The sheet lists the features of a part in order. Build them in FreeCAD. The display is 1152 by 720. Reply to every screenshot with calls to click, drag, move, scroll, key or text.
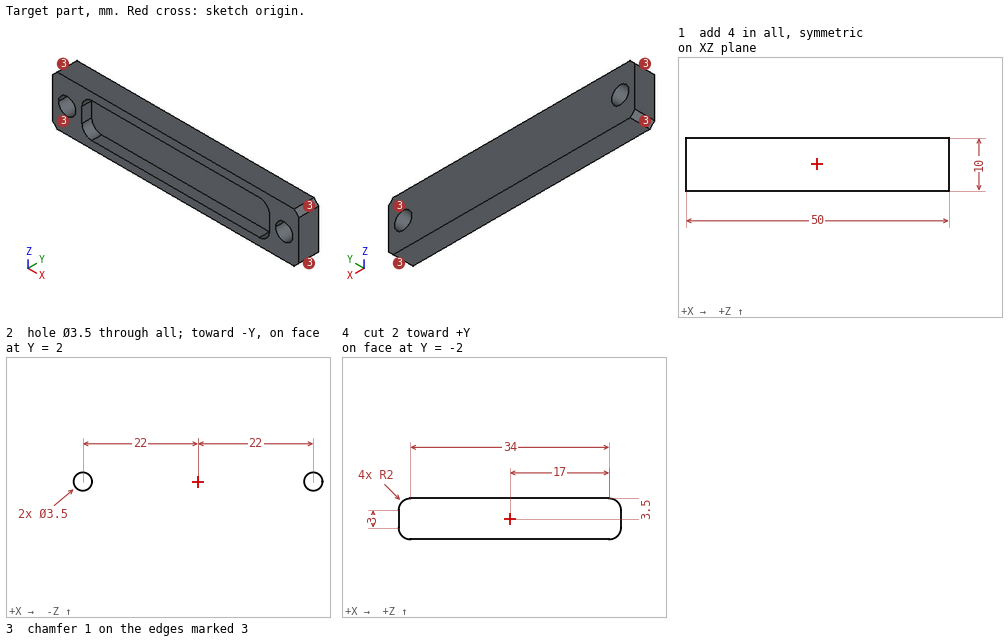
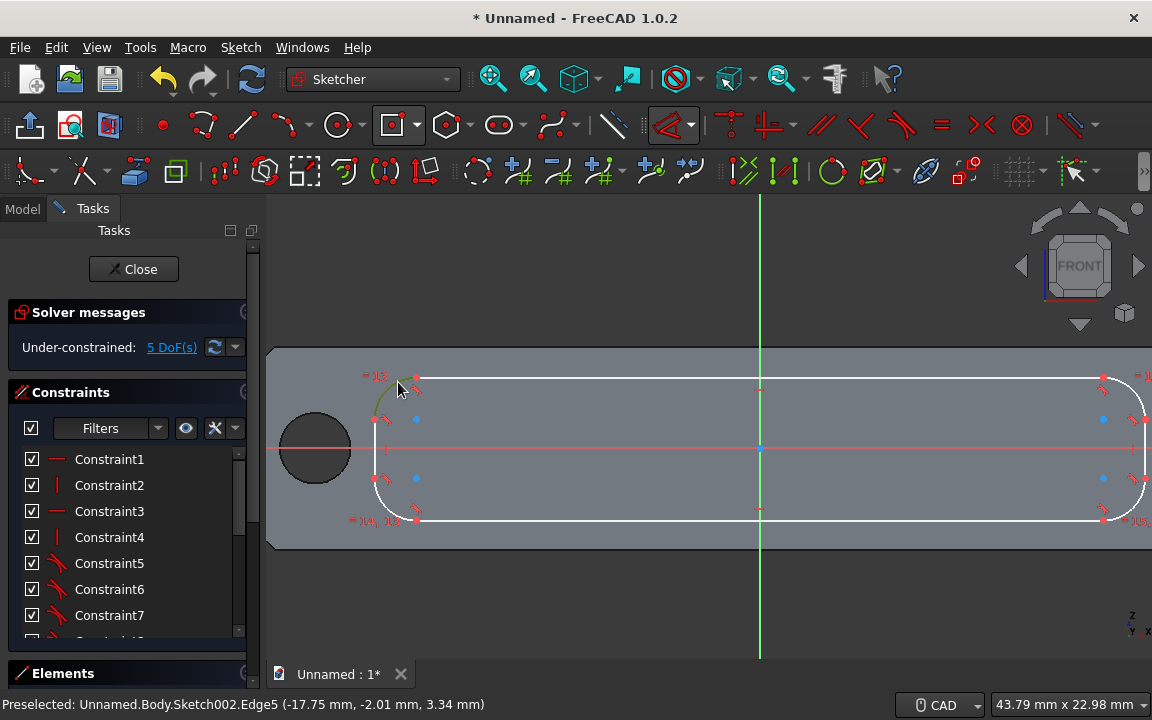
click(694, 126)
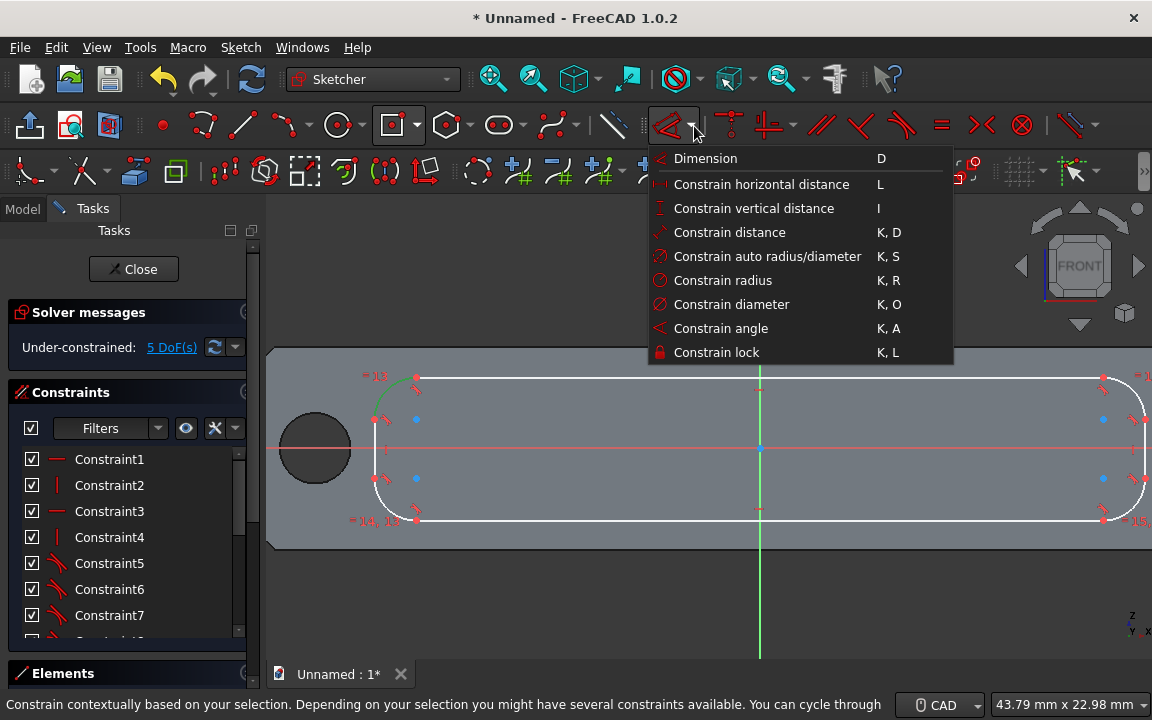
click(801, 280)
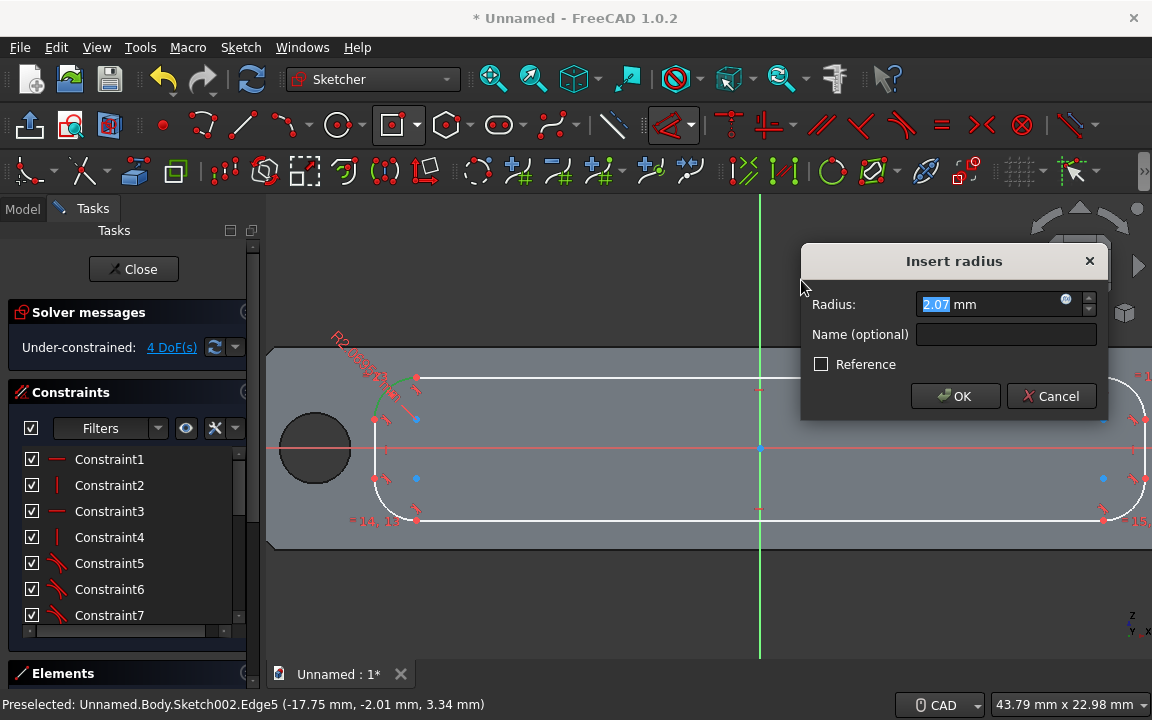
text(2)
key(Return)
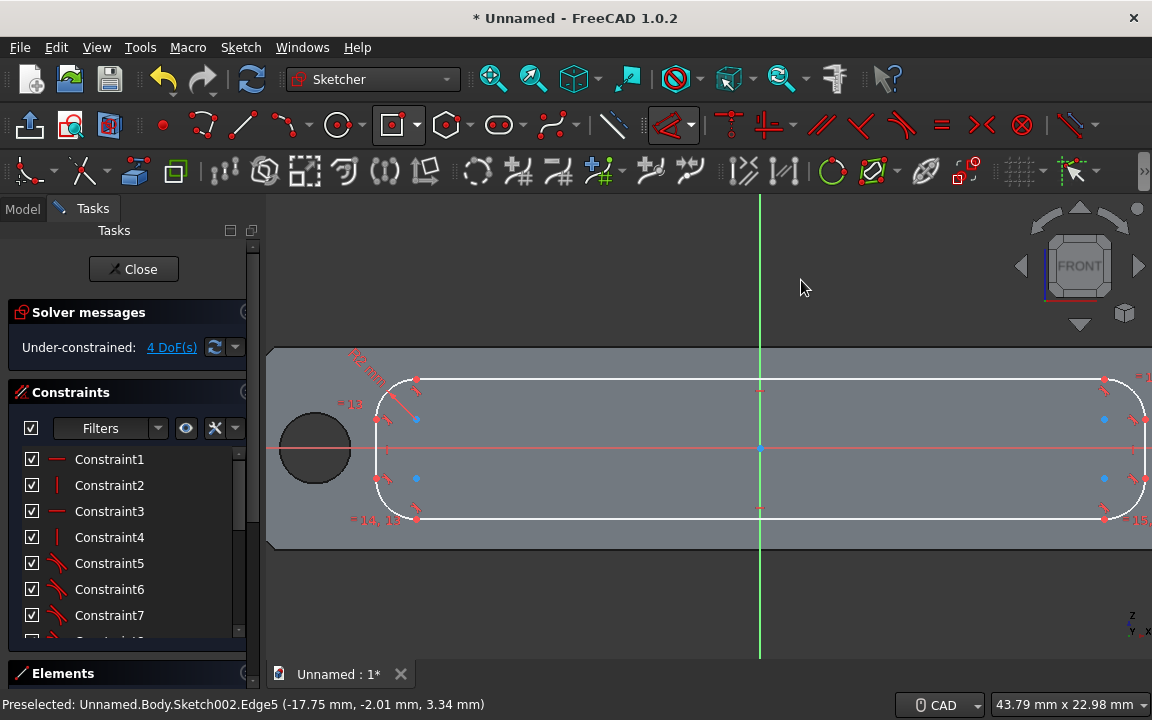
scroll(376, 437, up, 2)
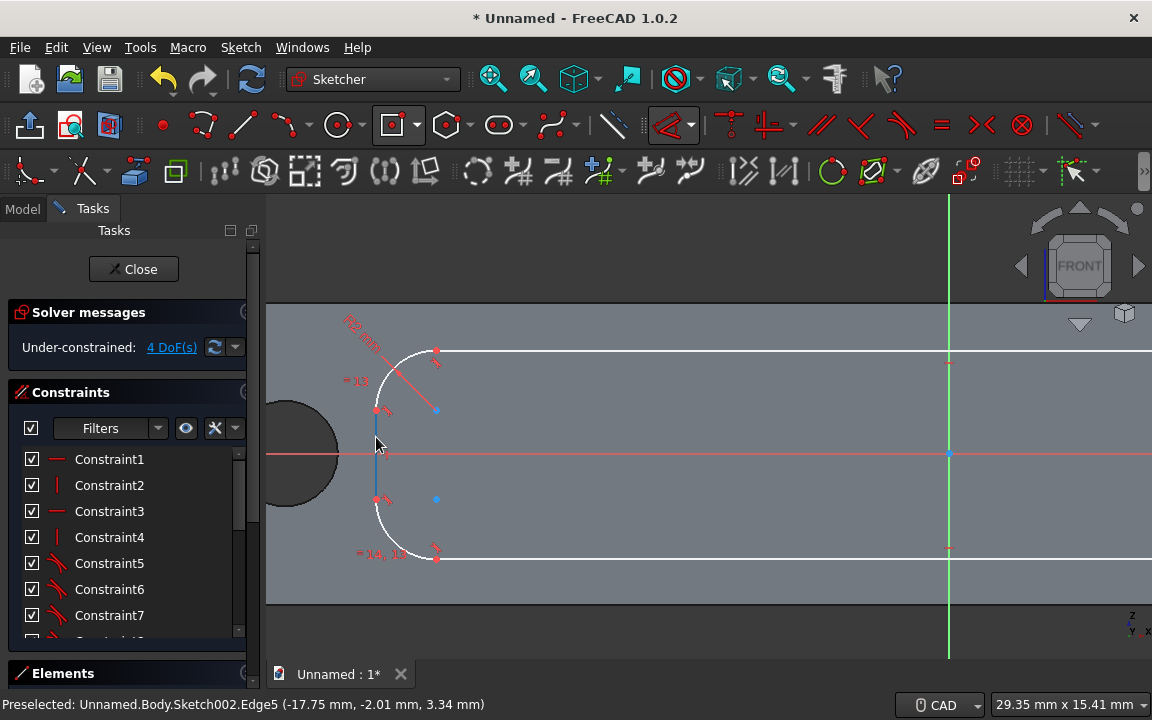
click(376, 437)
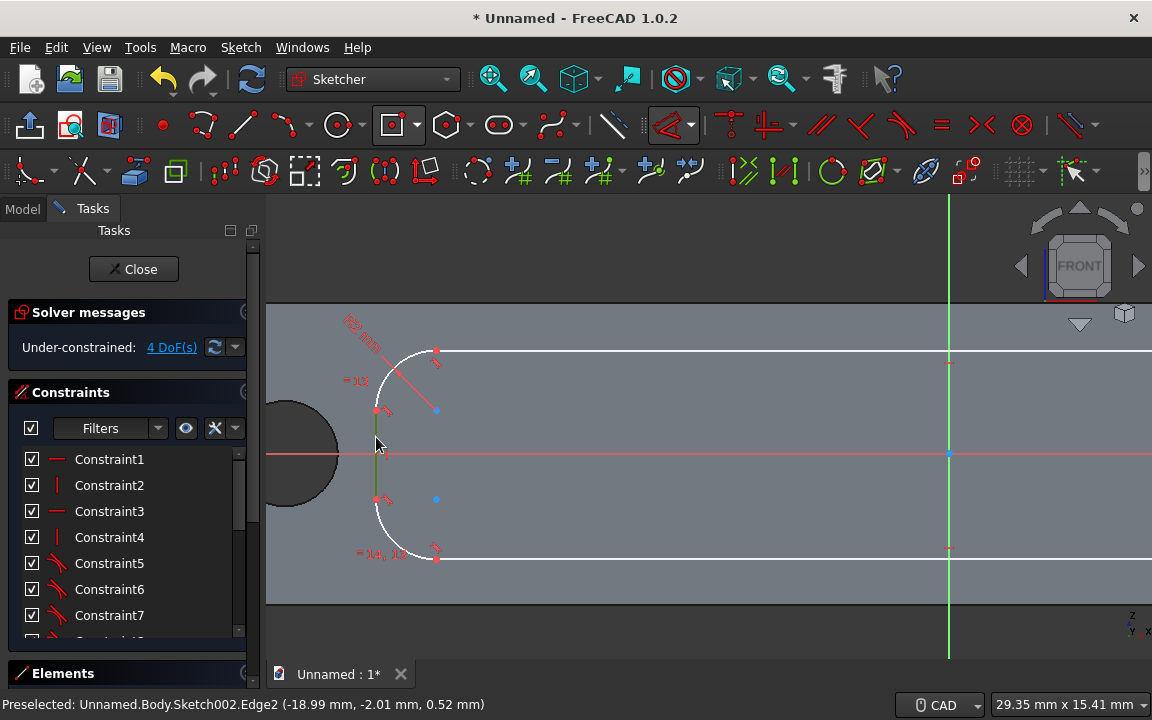
click(694, 126)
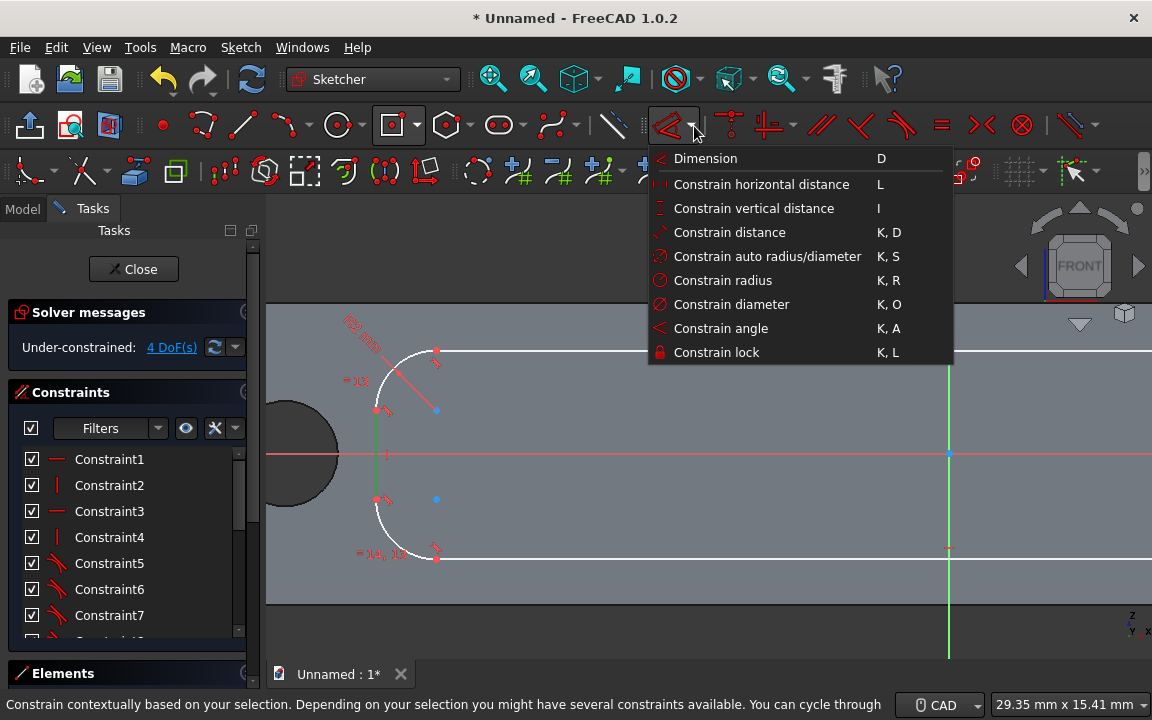
click(801, 208)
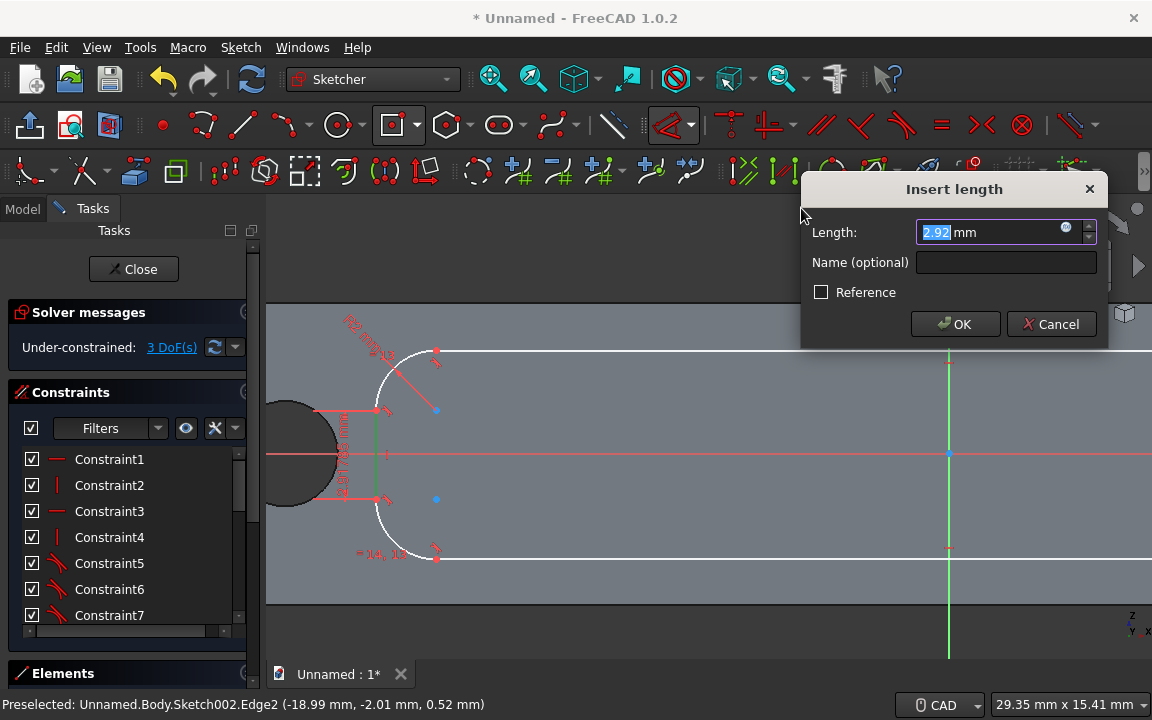
text(3)
key(Return)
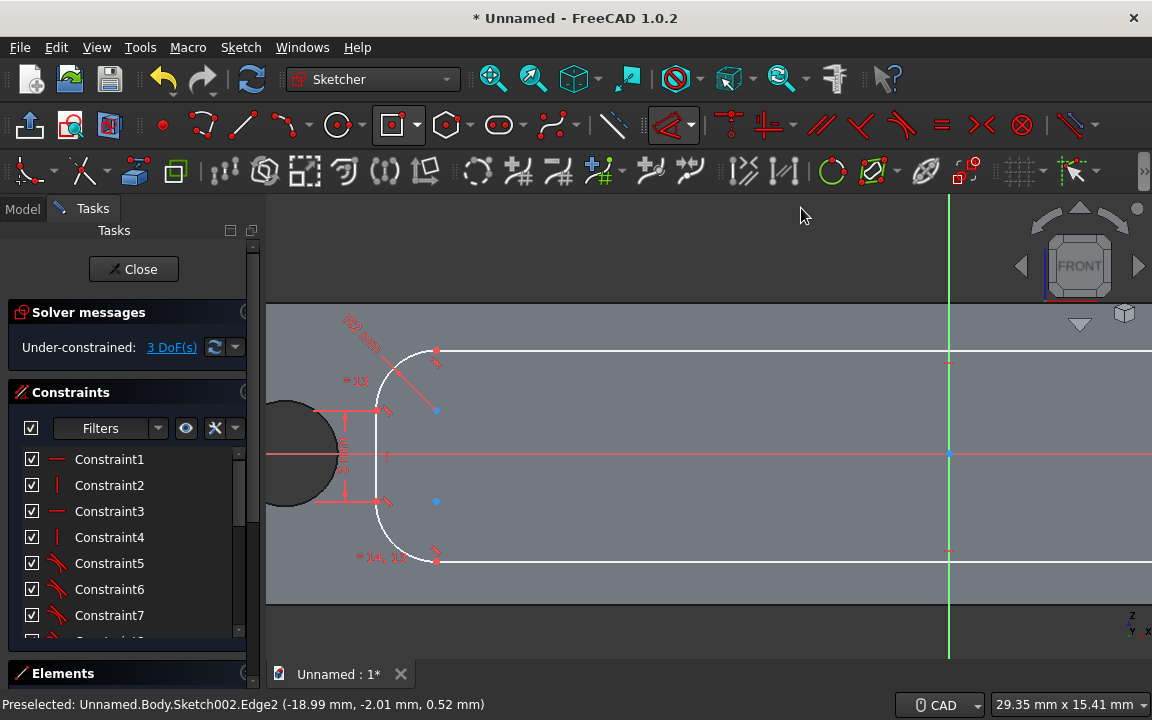
click(744, 351)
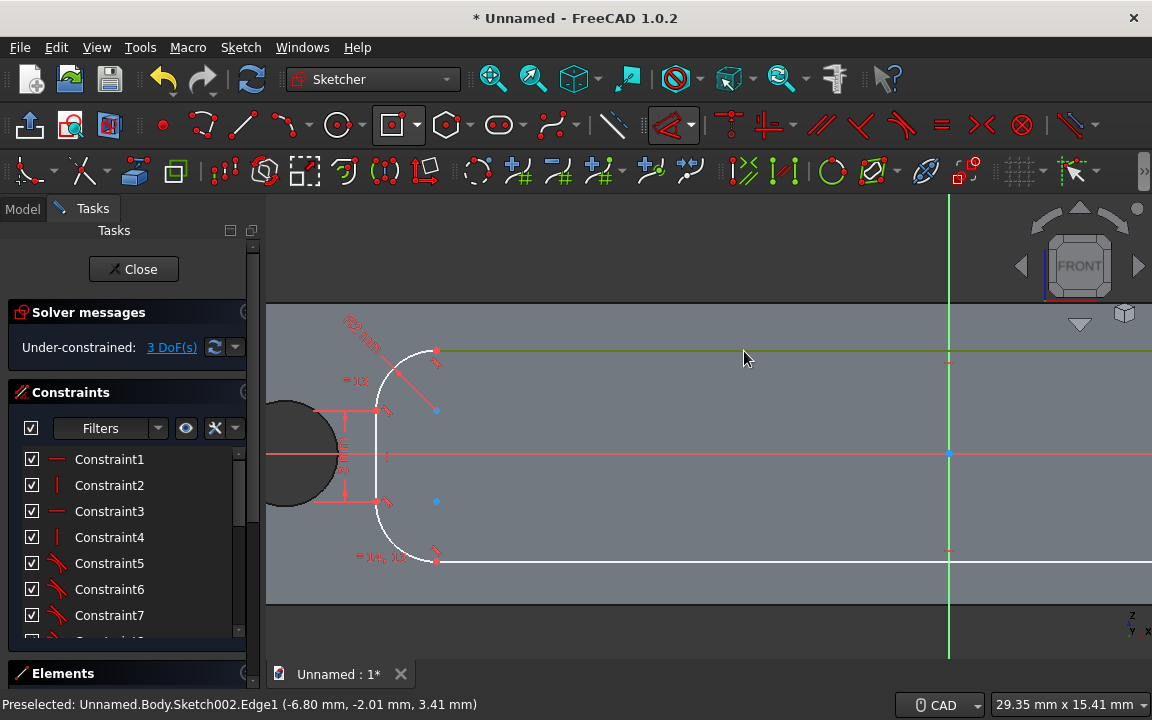
key(l)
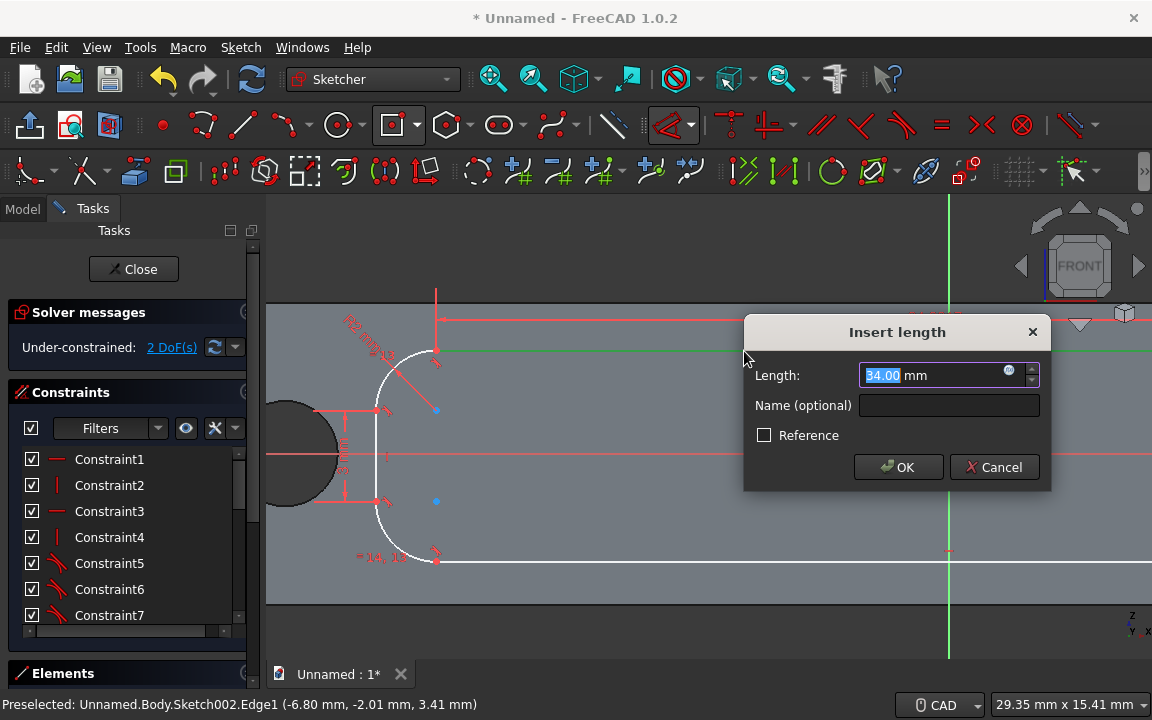
text(34)
key(Return)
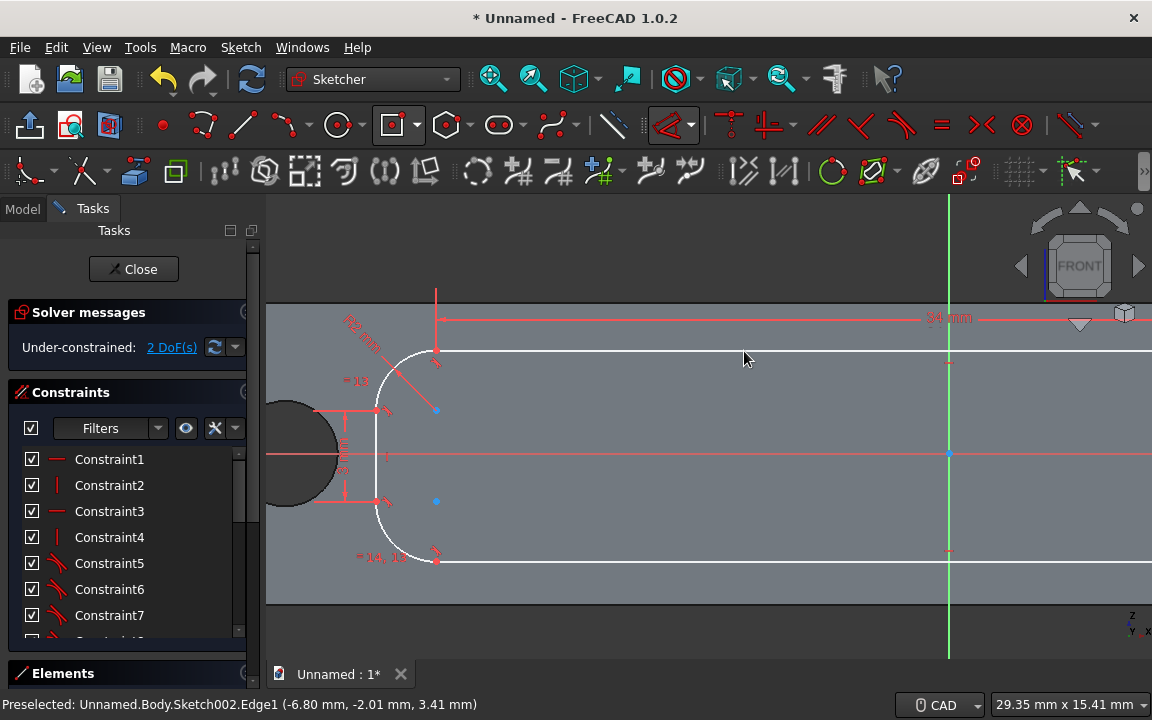
scroll(389, 404, down, 4)